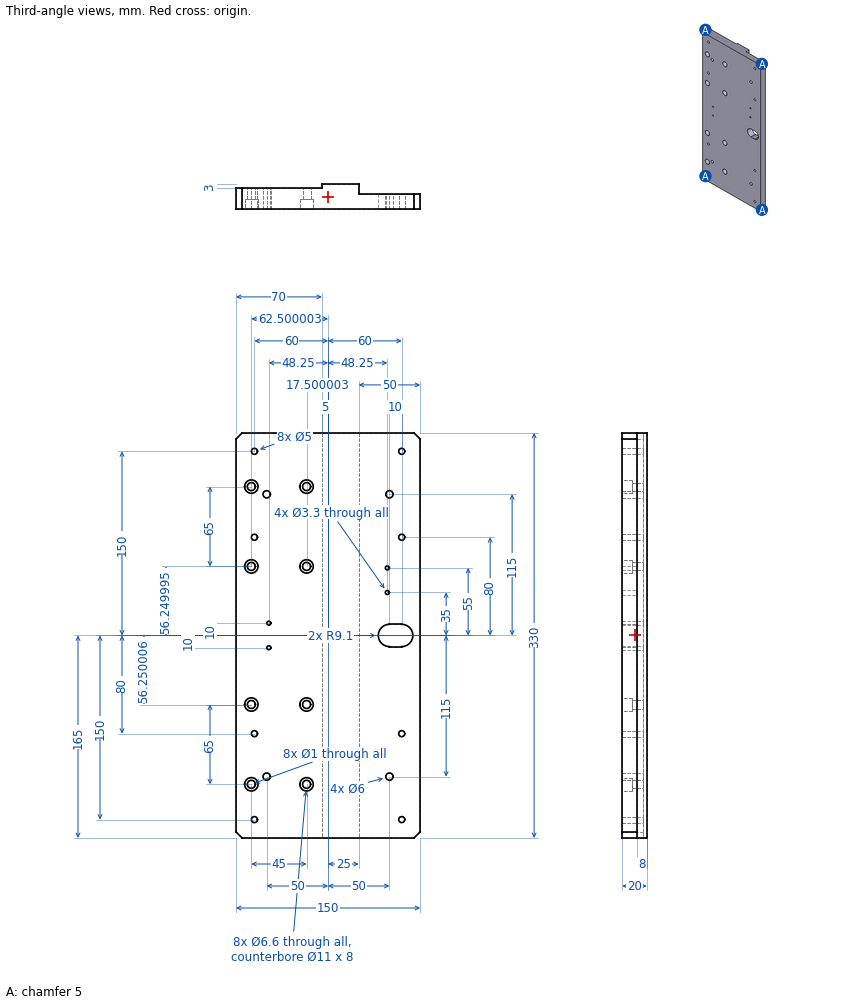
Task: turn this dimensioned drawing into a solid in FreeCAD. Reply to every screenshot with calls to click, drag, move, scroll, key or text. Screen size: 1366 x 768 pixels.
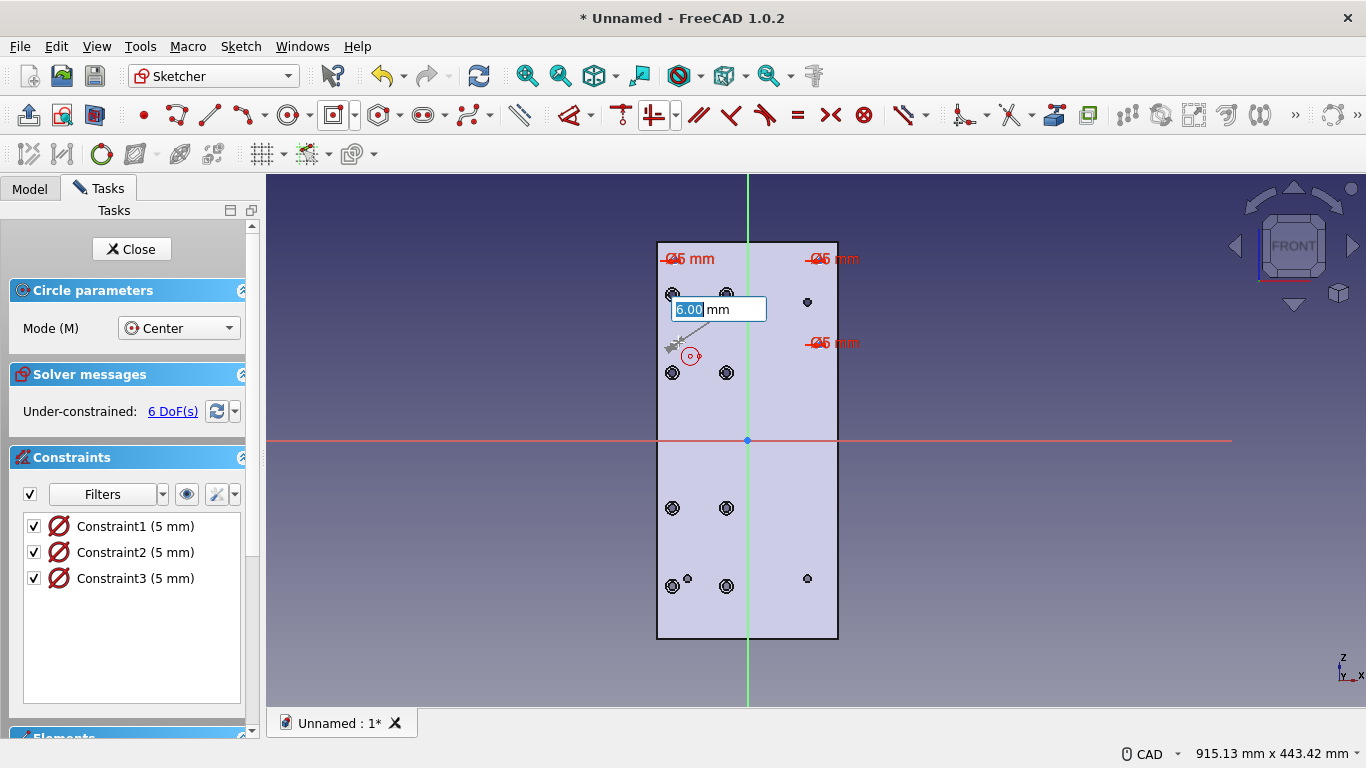
text(5)
key(Return)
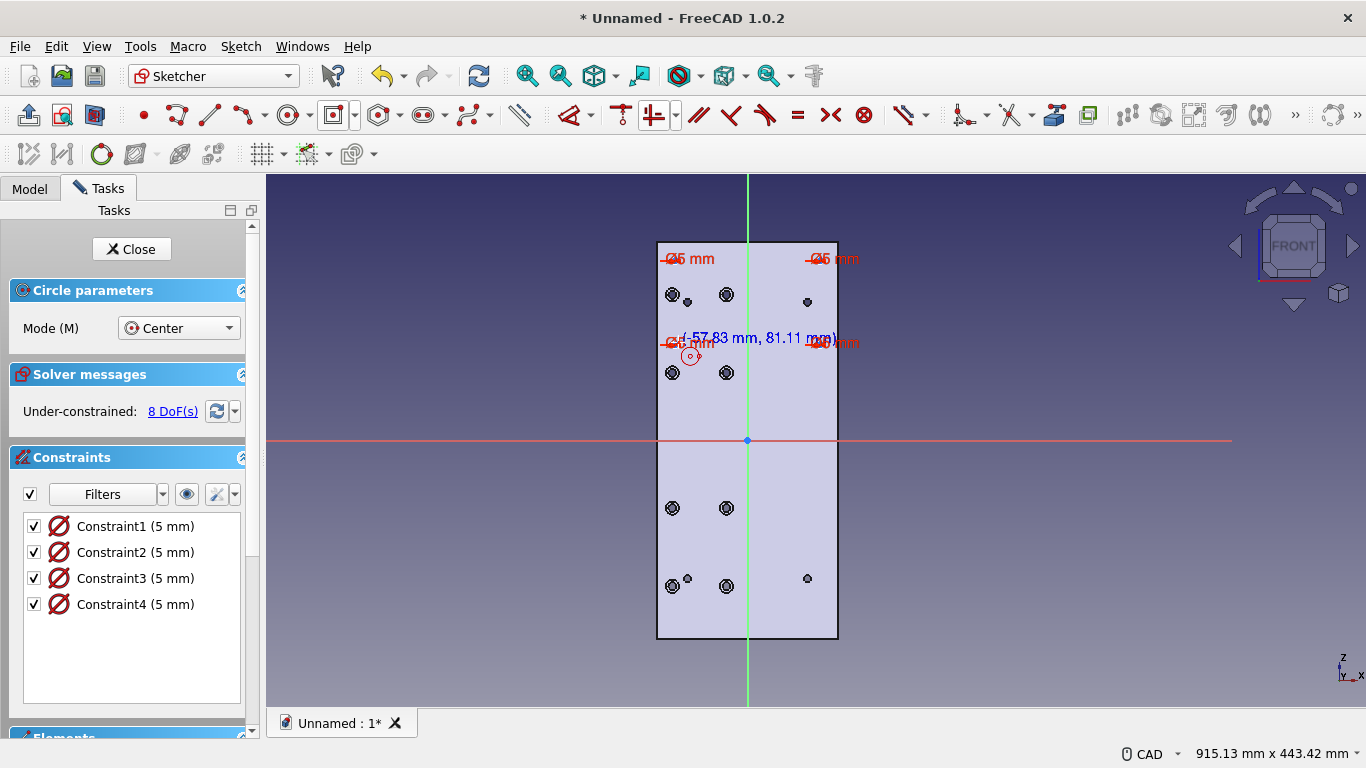
scroll(675, 537, up, 11)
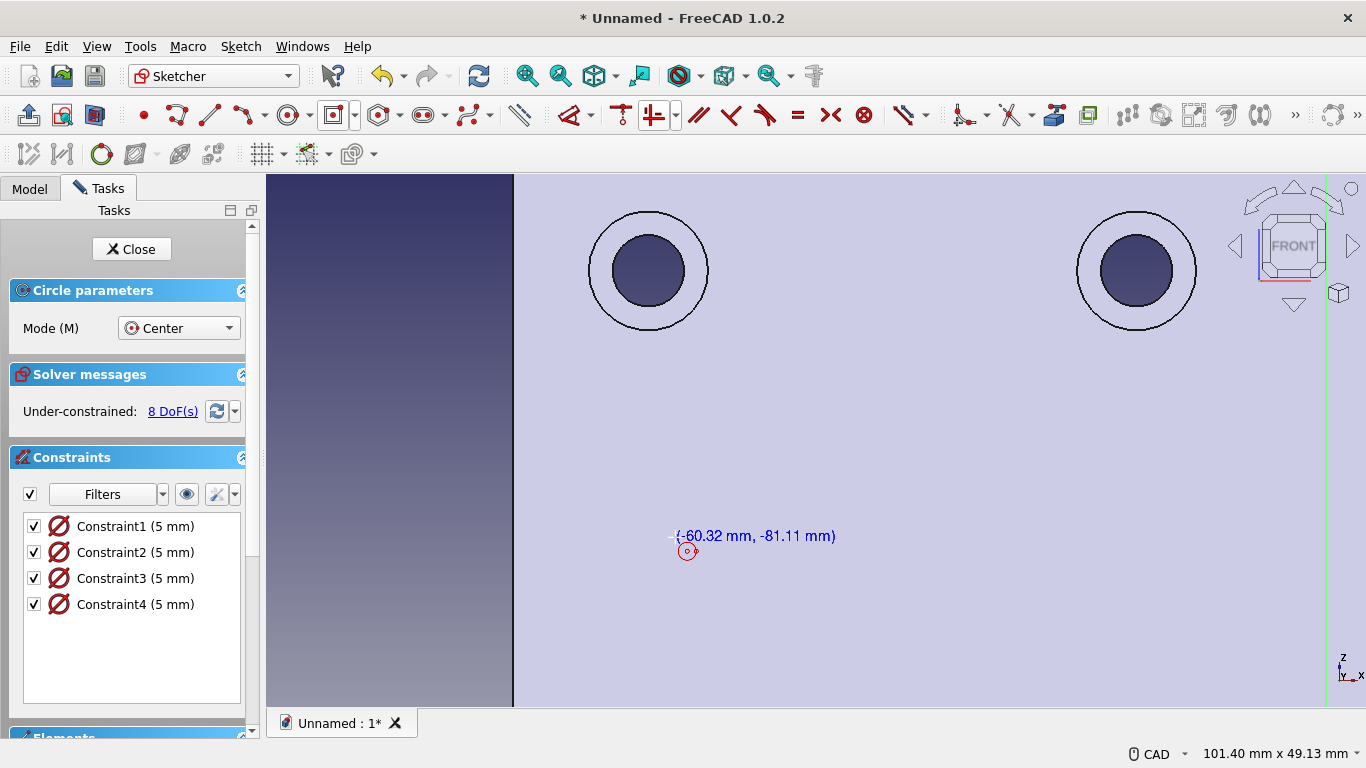
scroll(675, 538, down, 11)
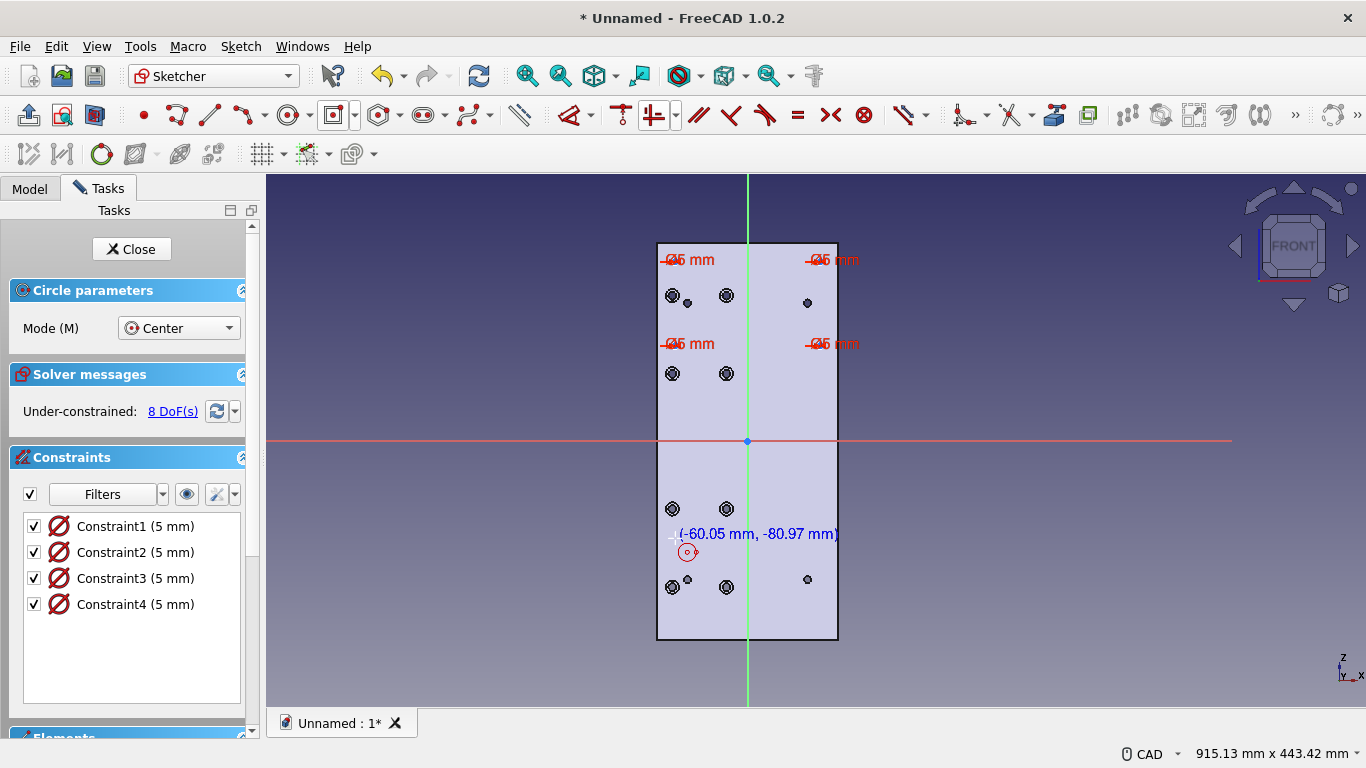
click(675, 538)
move(678, 535)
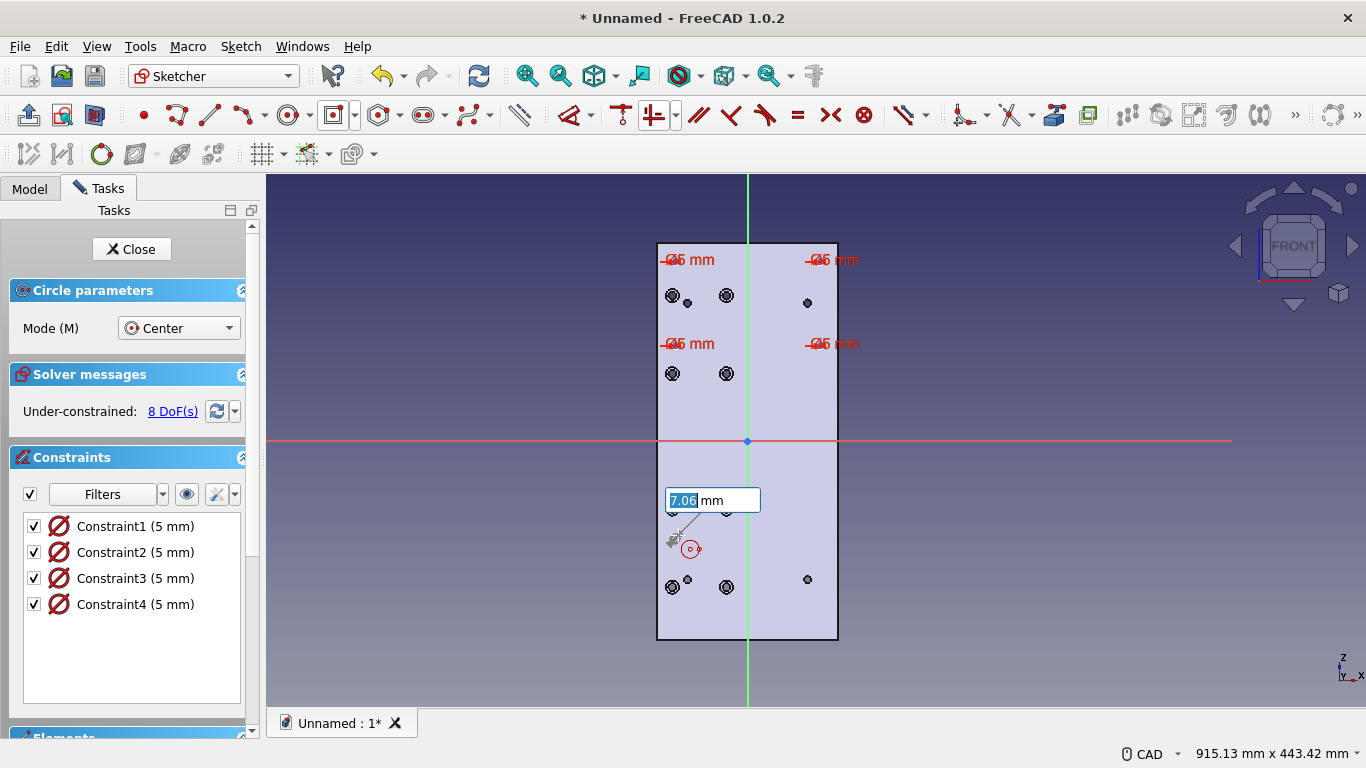
text(5)
key(Return)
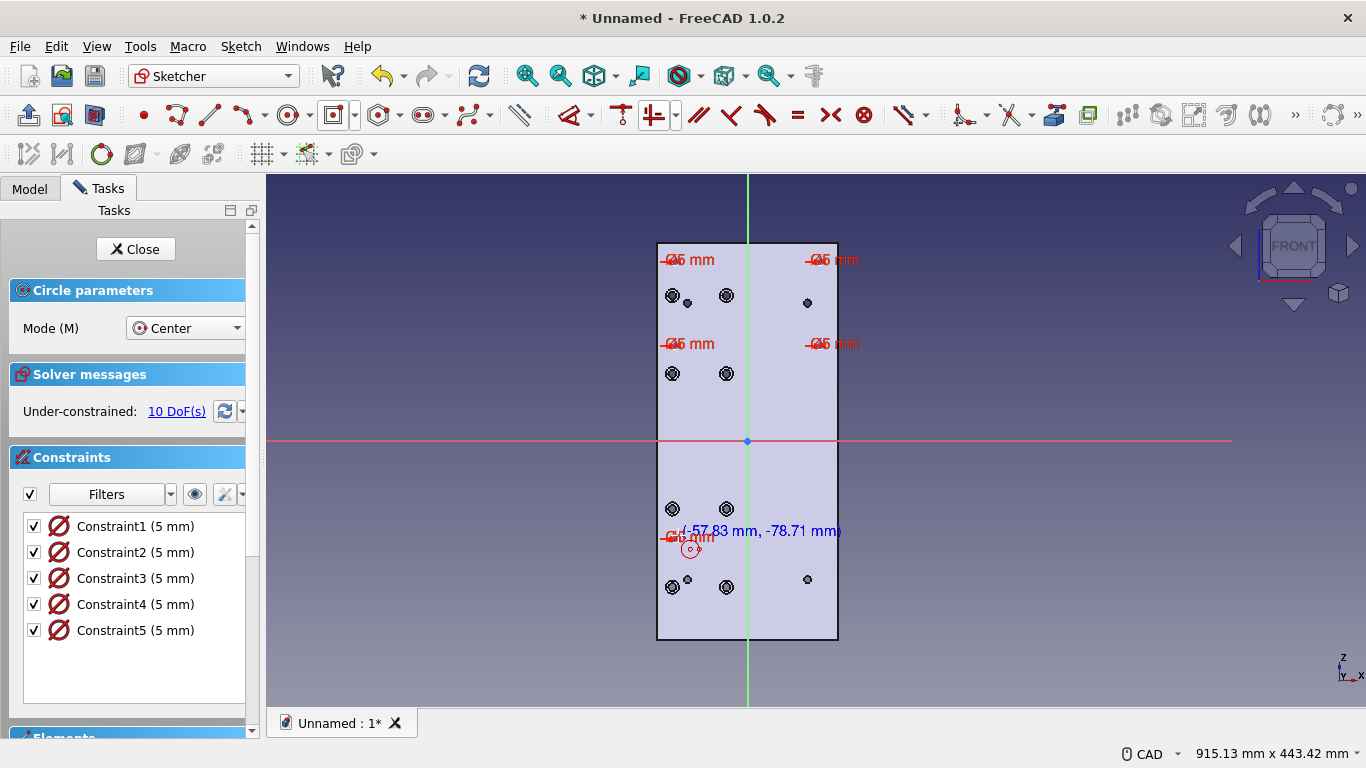
scroll(675, 622, up, 11)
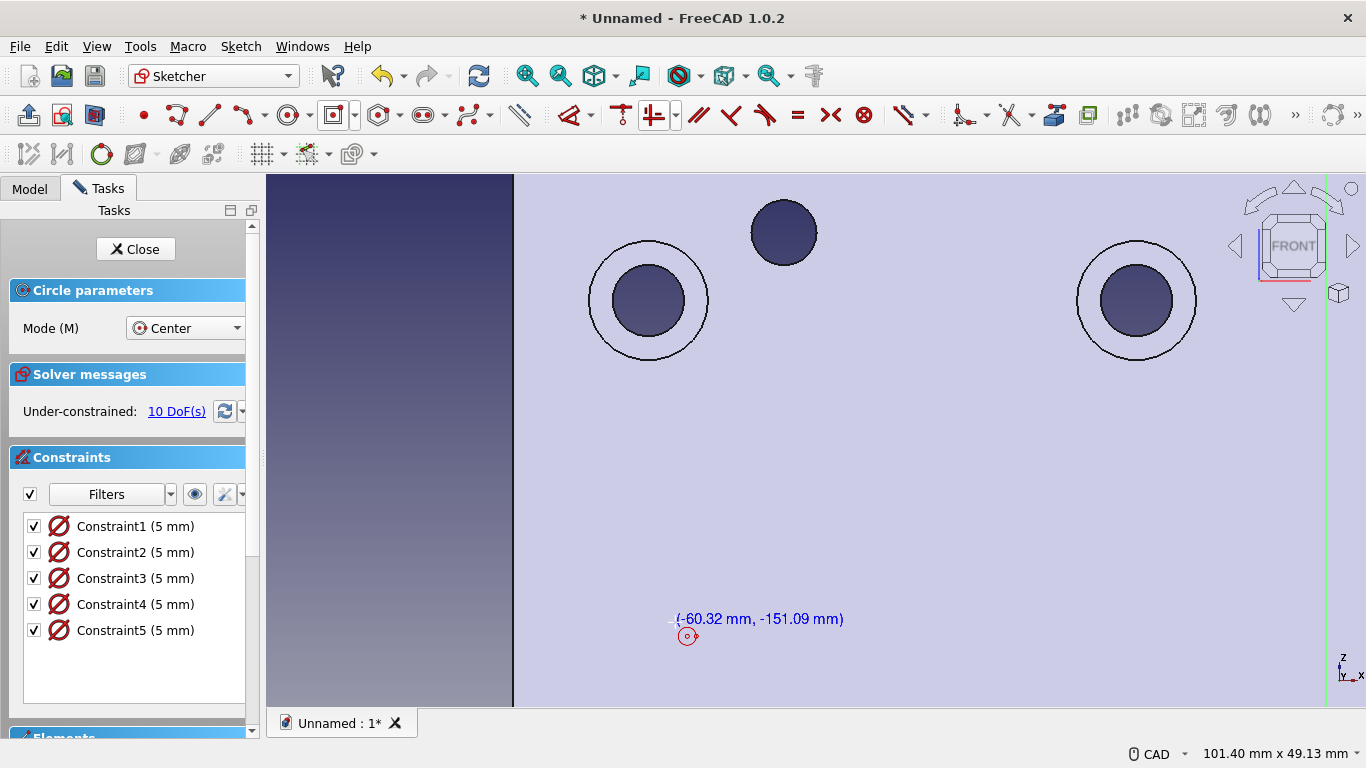
scroll(675, 622, down, 11)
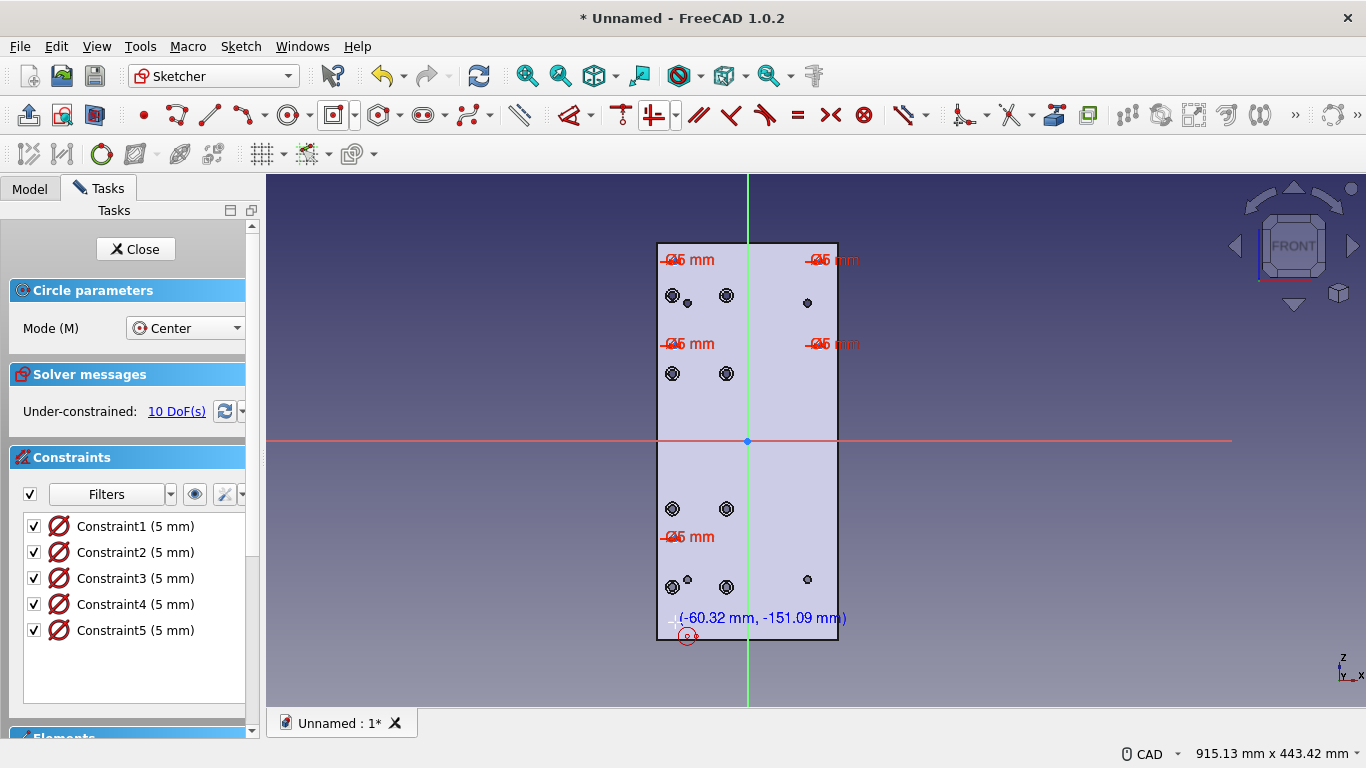
click(675, 622)
move(678, 620)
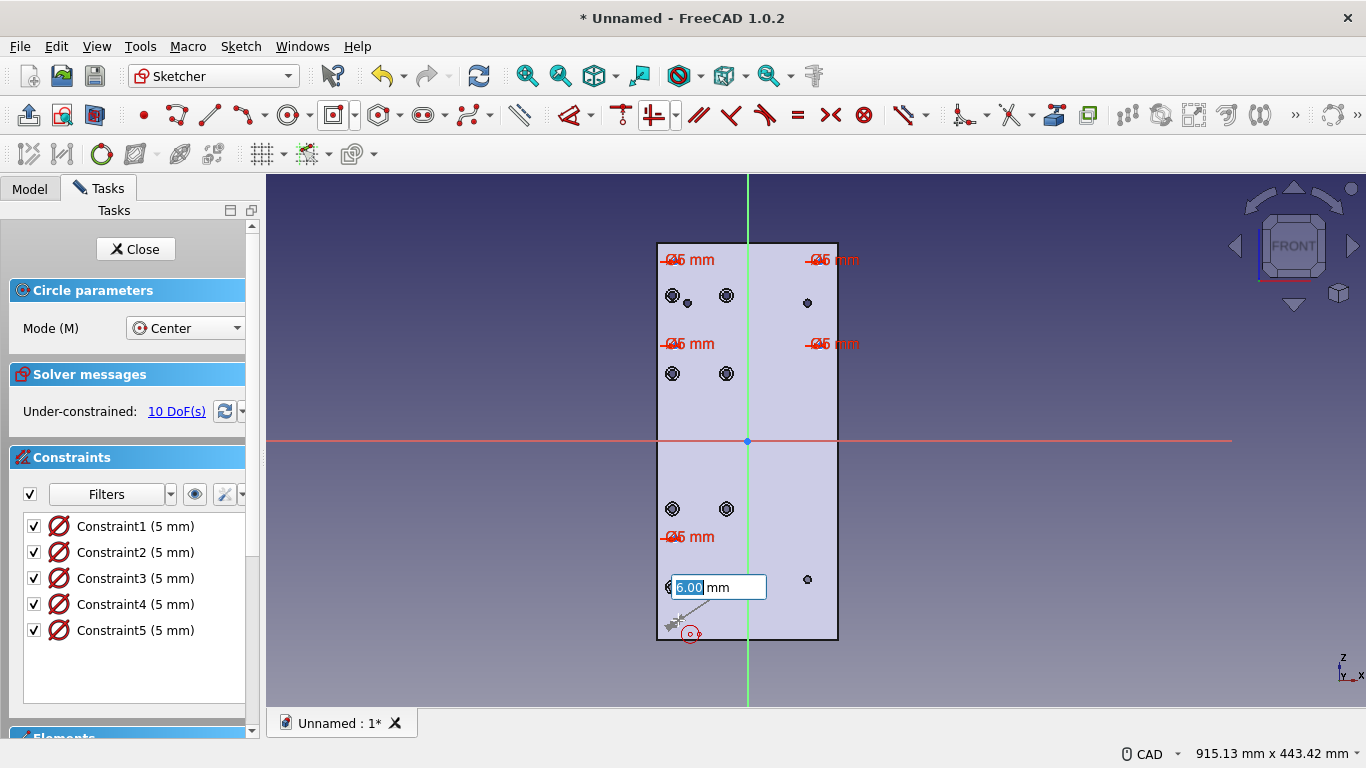
text(5)
key(Return)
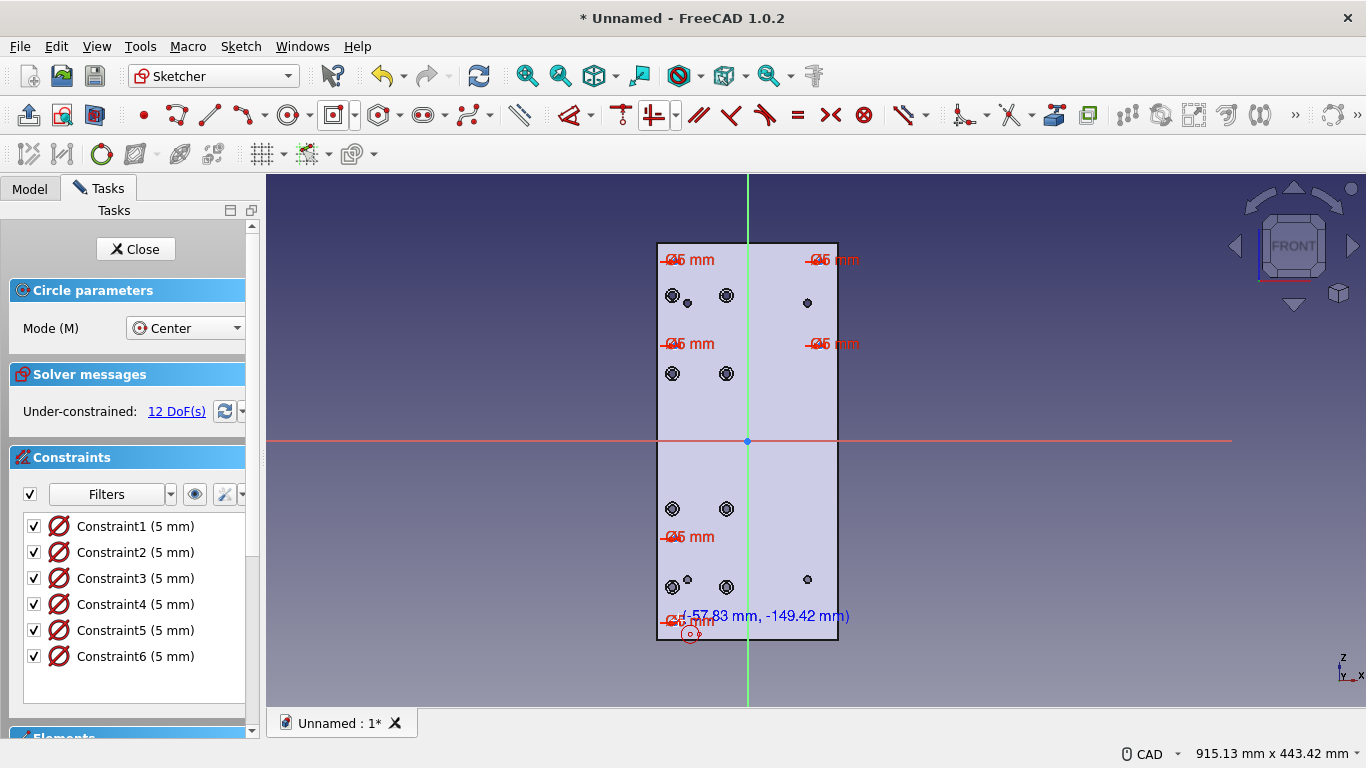
scroll(820, 622, up, 11)